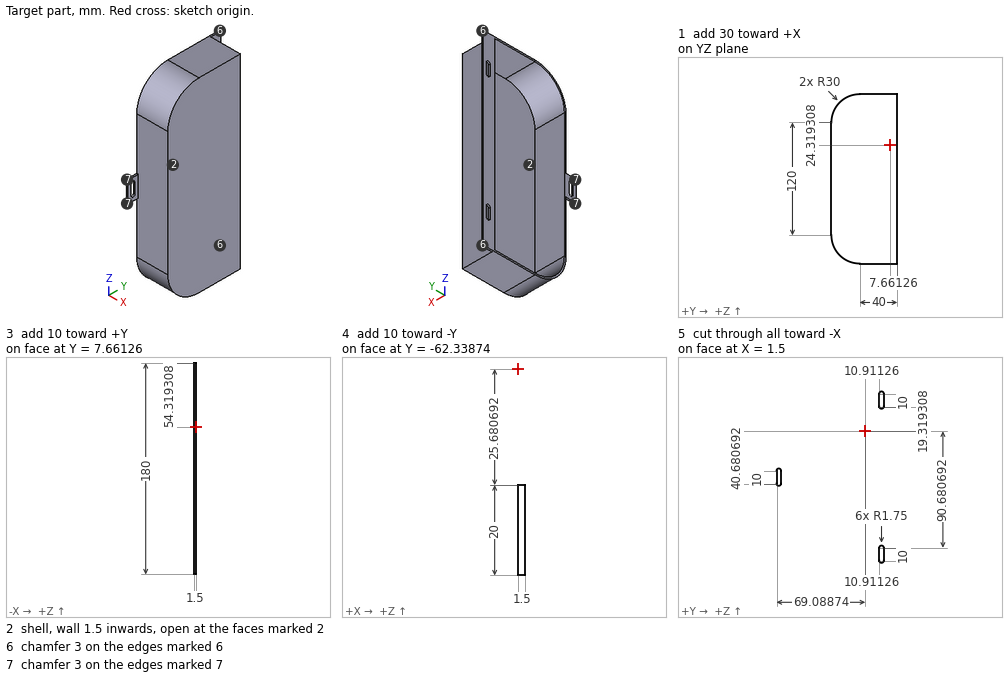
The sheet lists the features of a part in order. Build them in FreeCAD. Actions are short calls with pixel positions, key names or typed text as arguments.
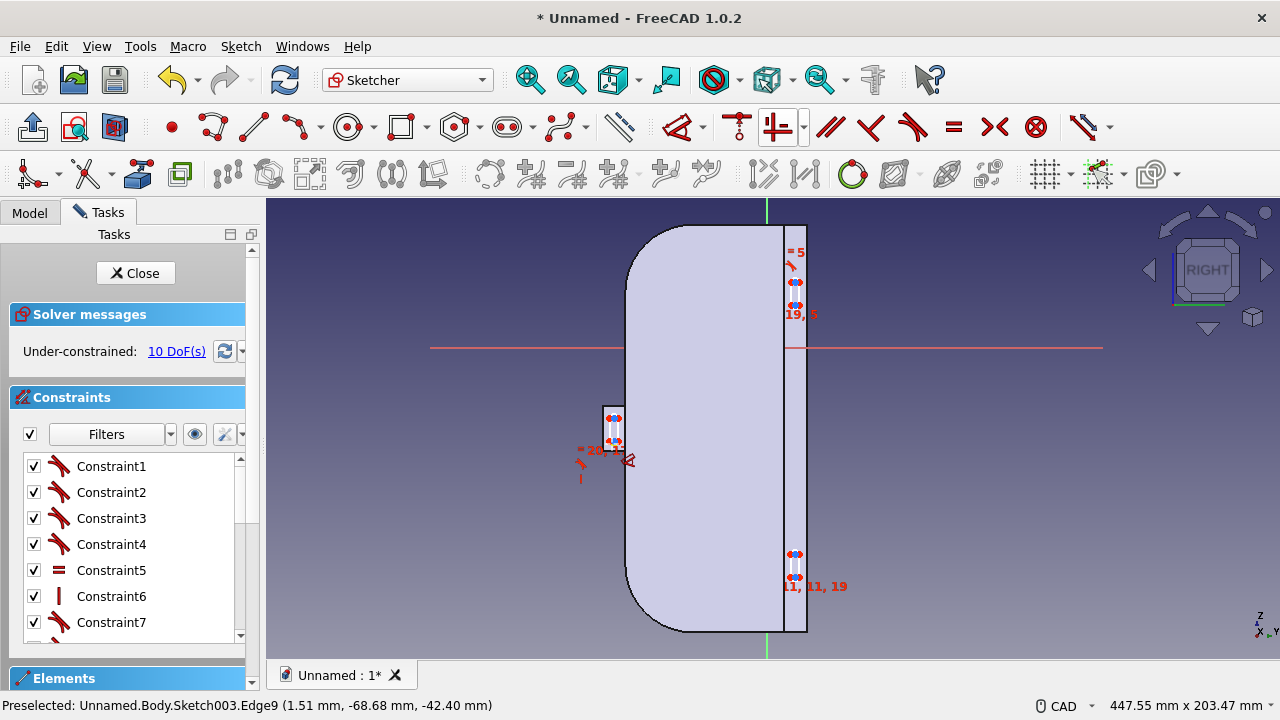
scroll(793, 308, up, 12)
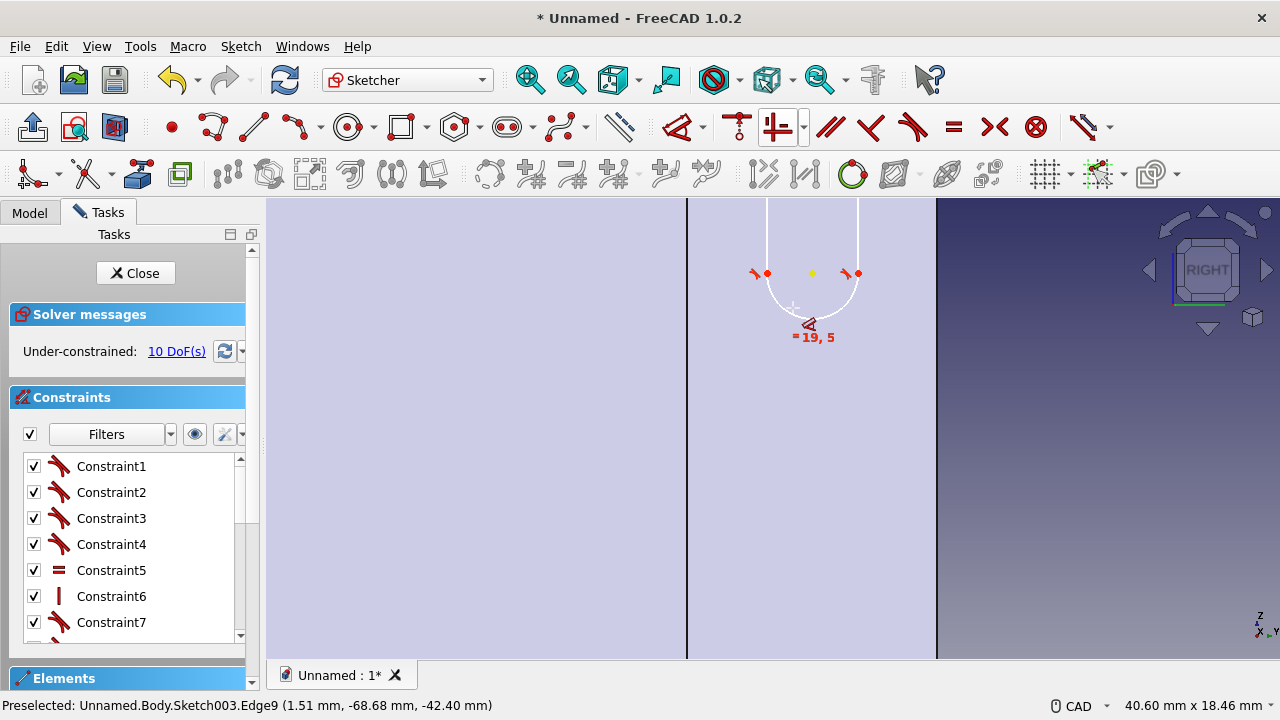
click(786, 310)
click(767, 336)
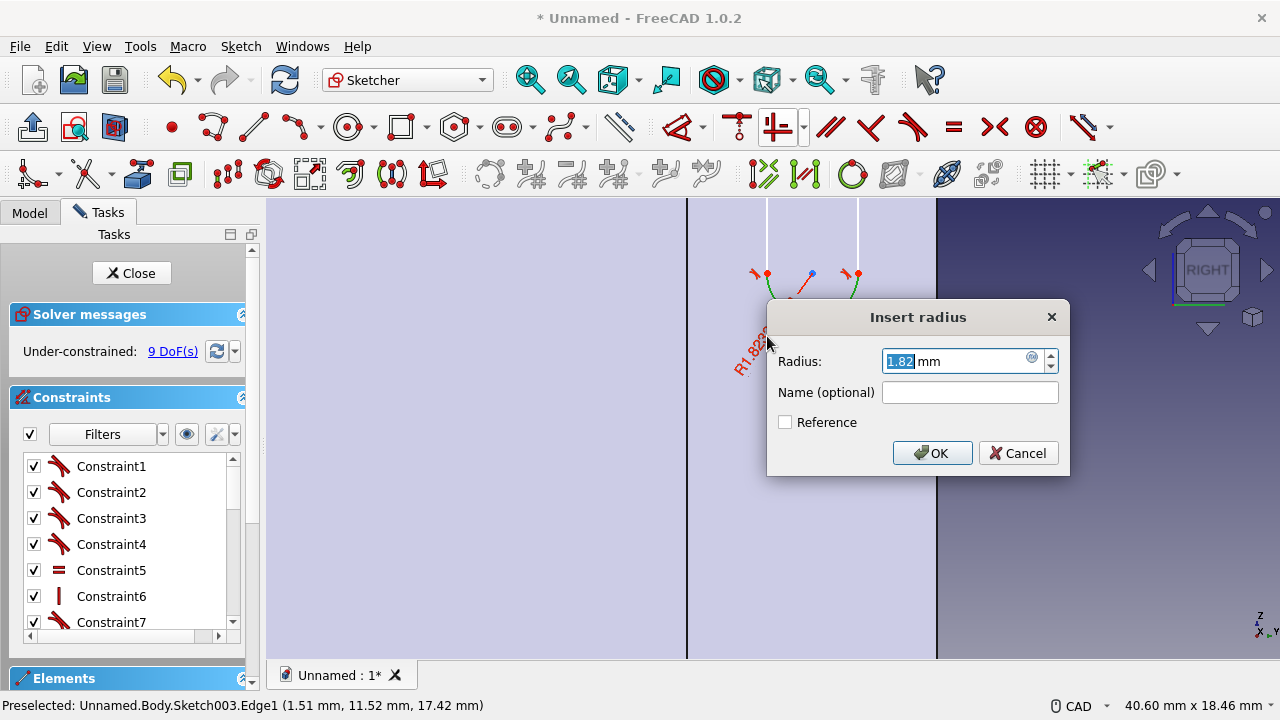
text(1.75)
key(Return)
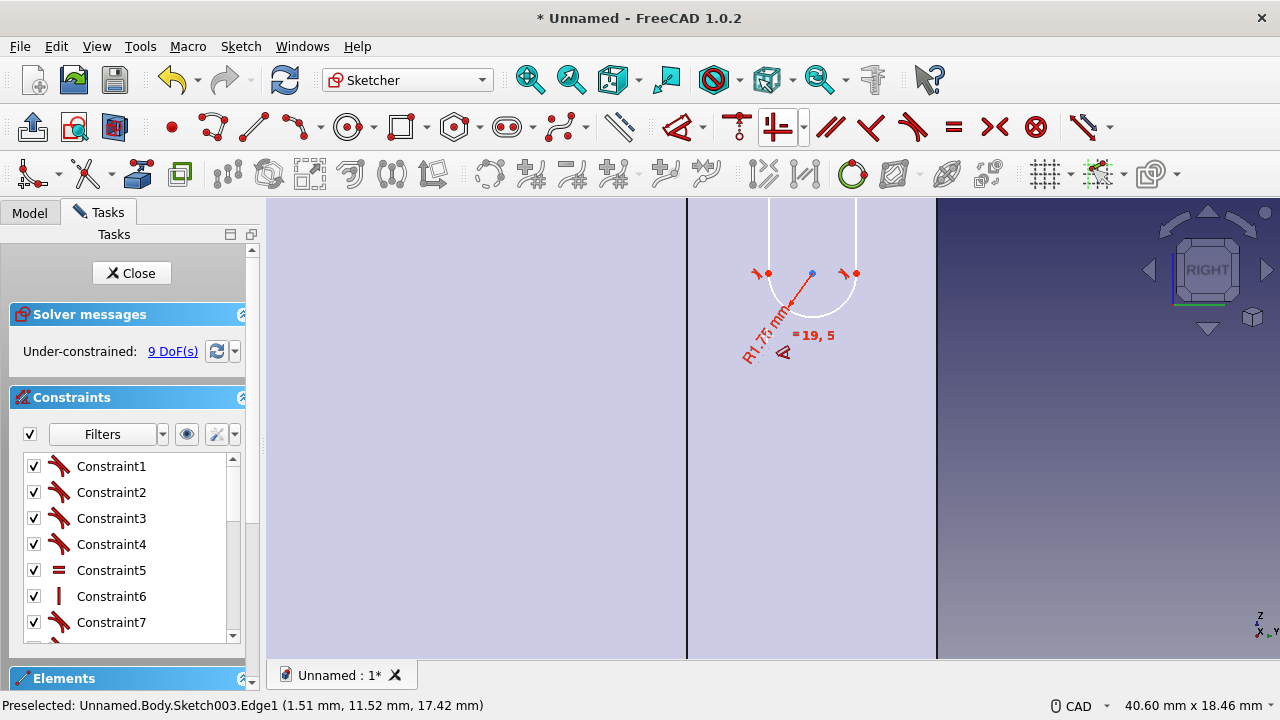
scroll(793, 308, down, 12)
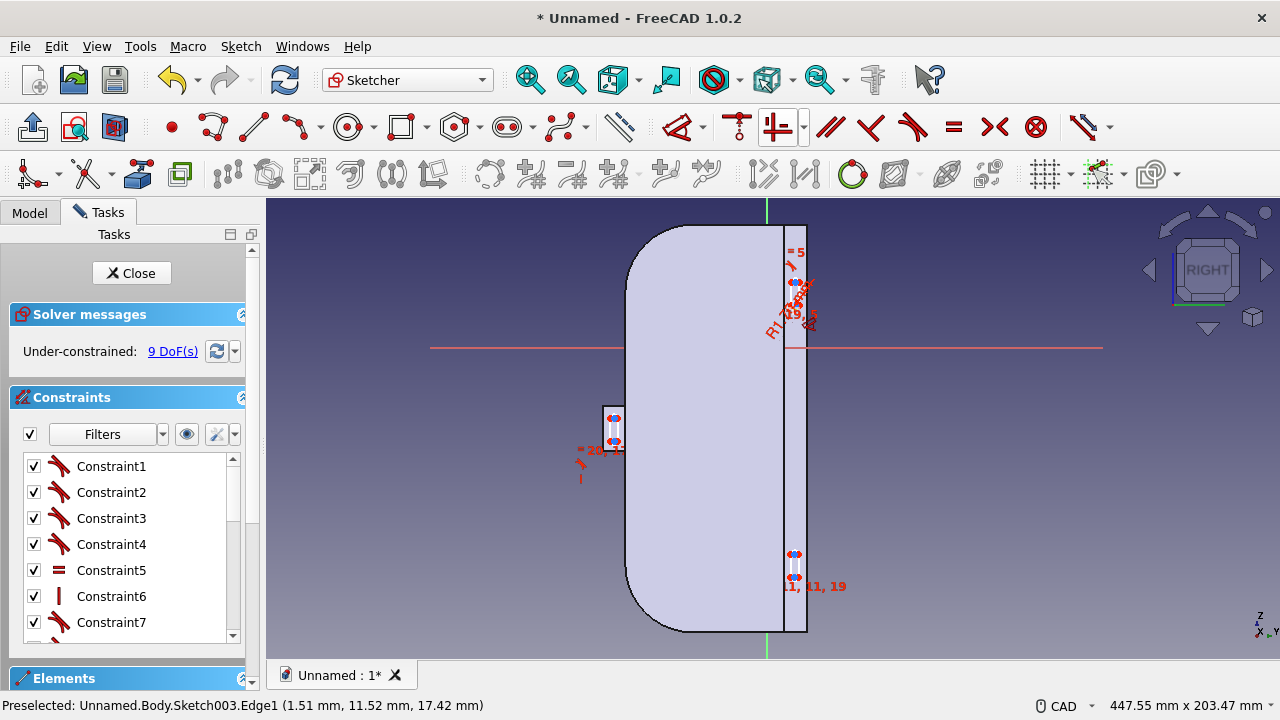
scroll(791, 298, up, 4)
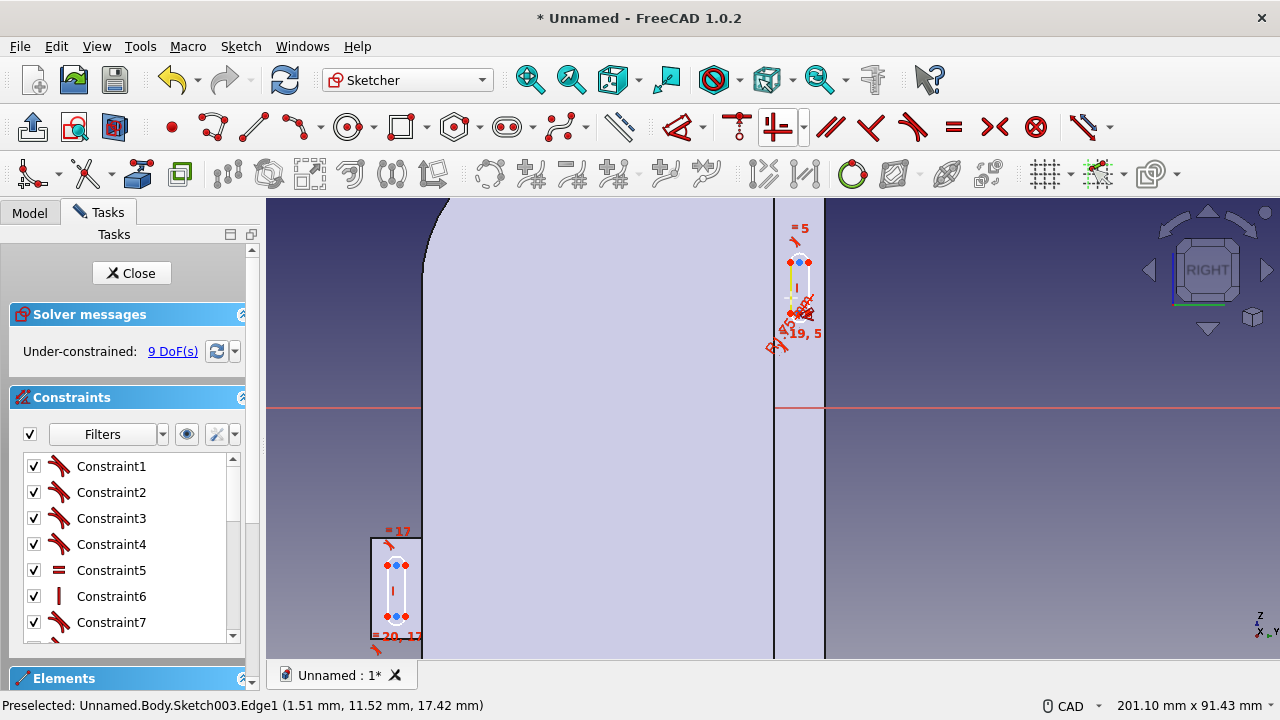
click(791, 298)
click(825, 288)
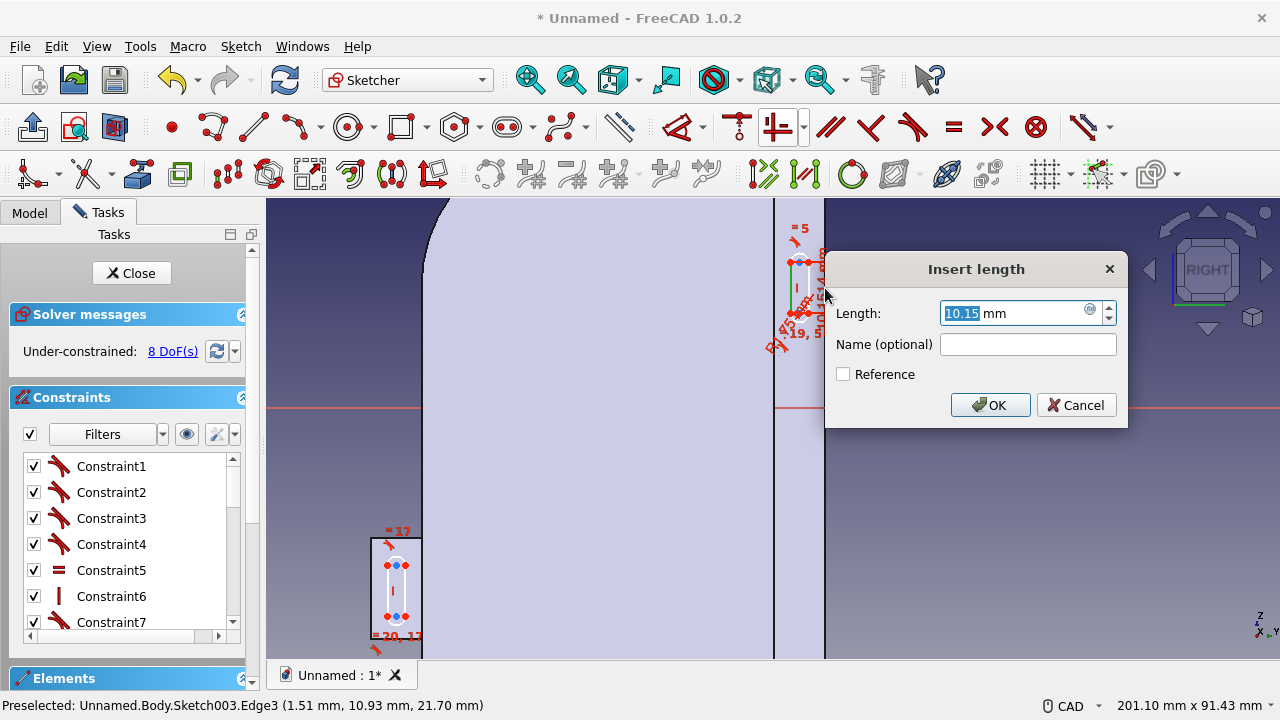
text(10)
key(Return)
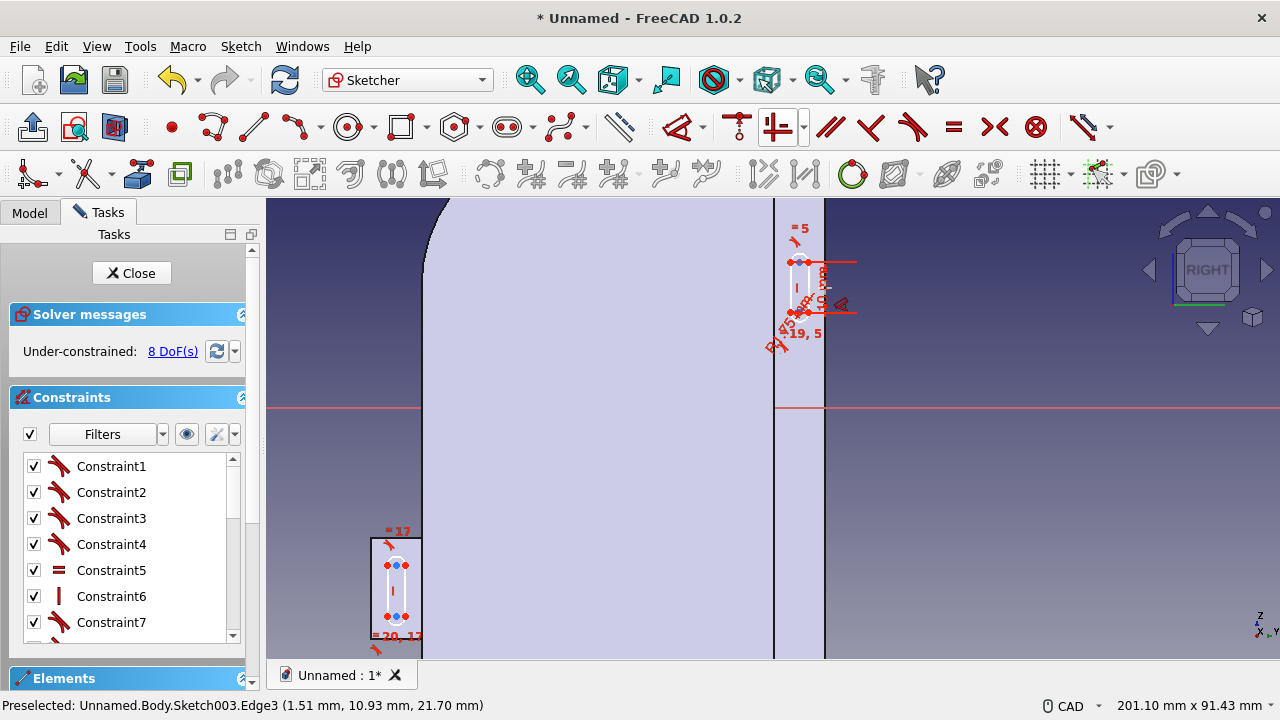
scroll(791, 298, down, 4)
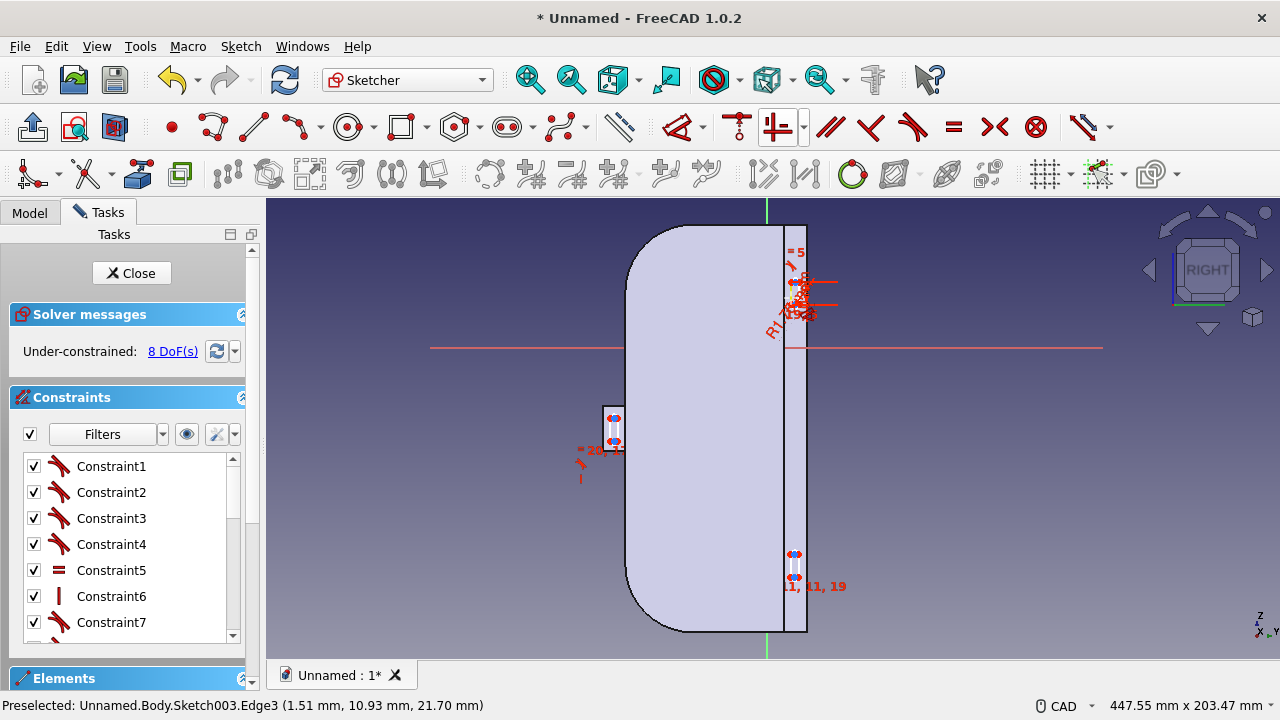
scroll(791, 570, up, 4)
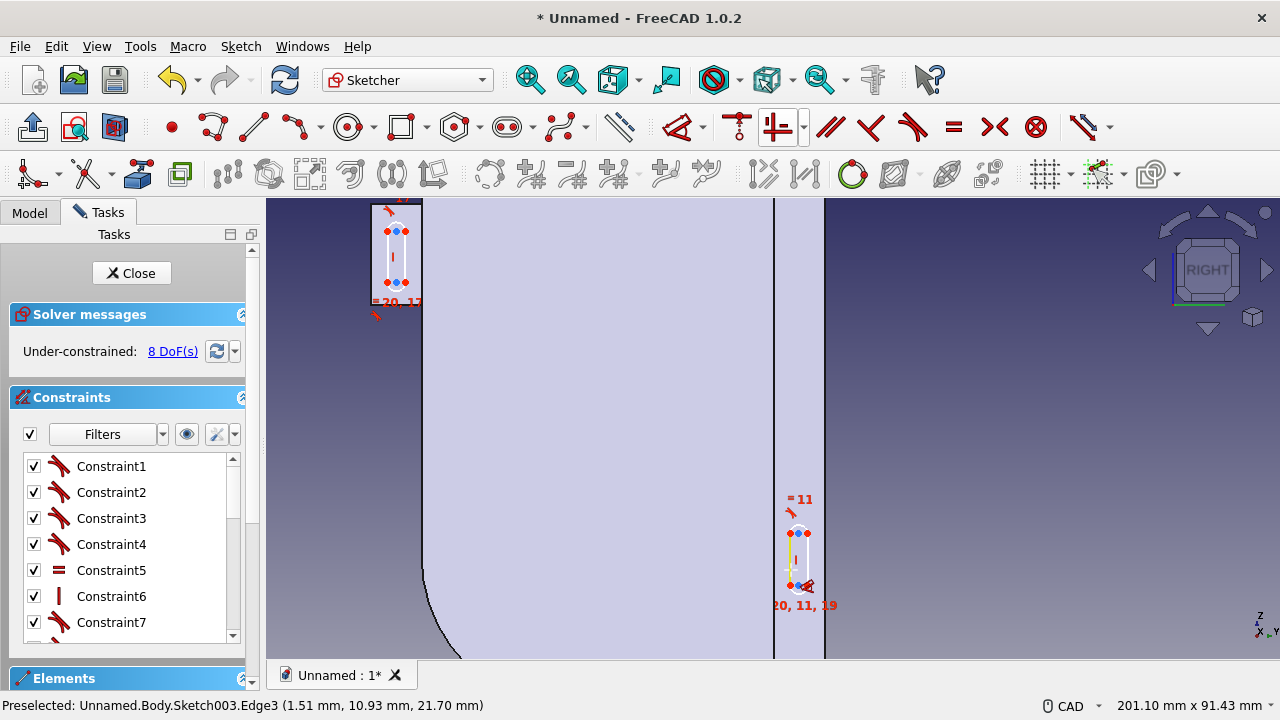
click(790, 570)
click(824, 560)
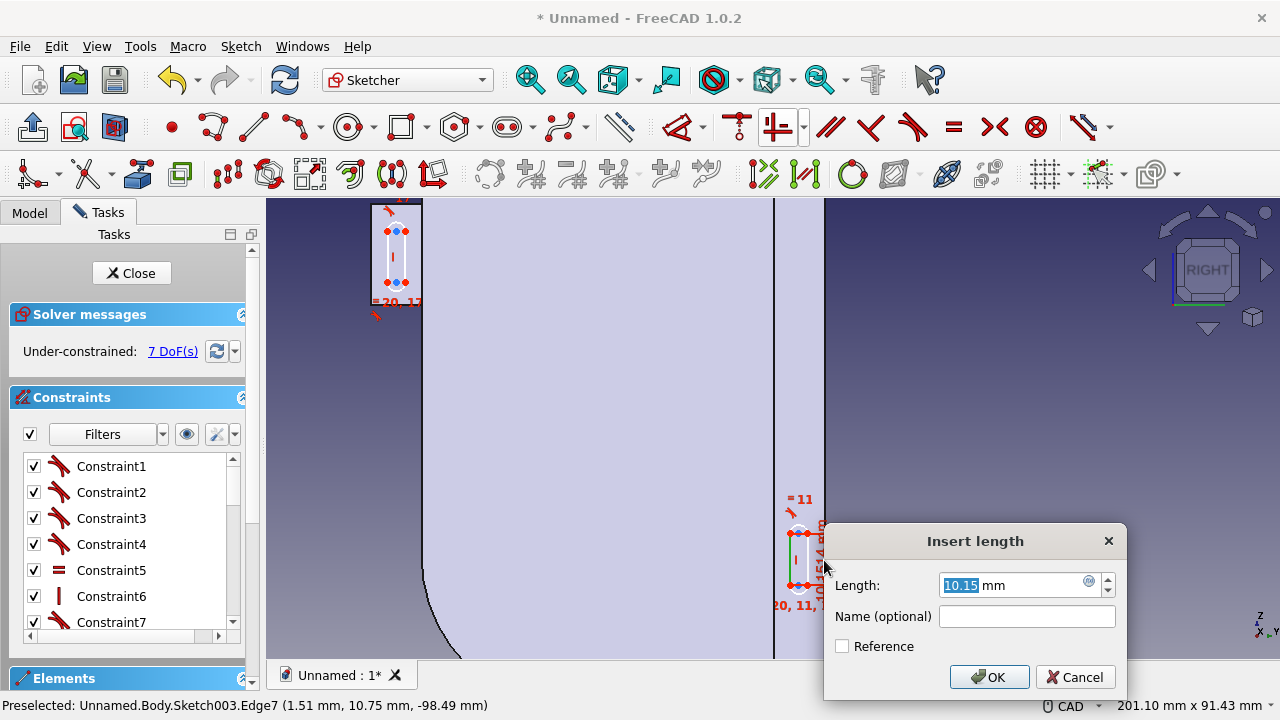
text(10)
key(Return)